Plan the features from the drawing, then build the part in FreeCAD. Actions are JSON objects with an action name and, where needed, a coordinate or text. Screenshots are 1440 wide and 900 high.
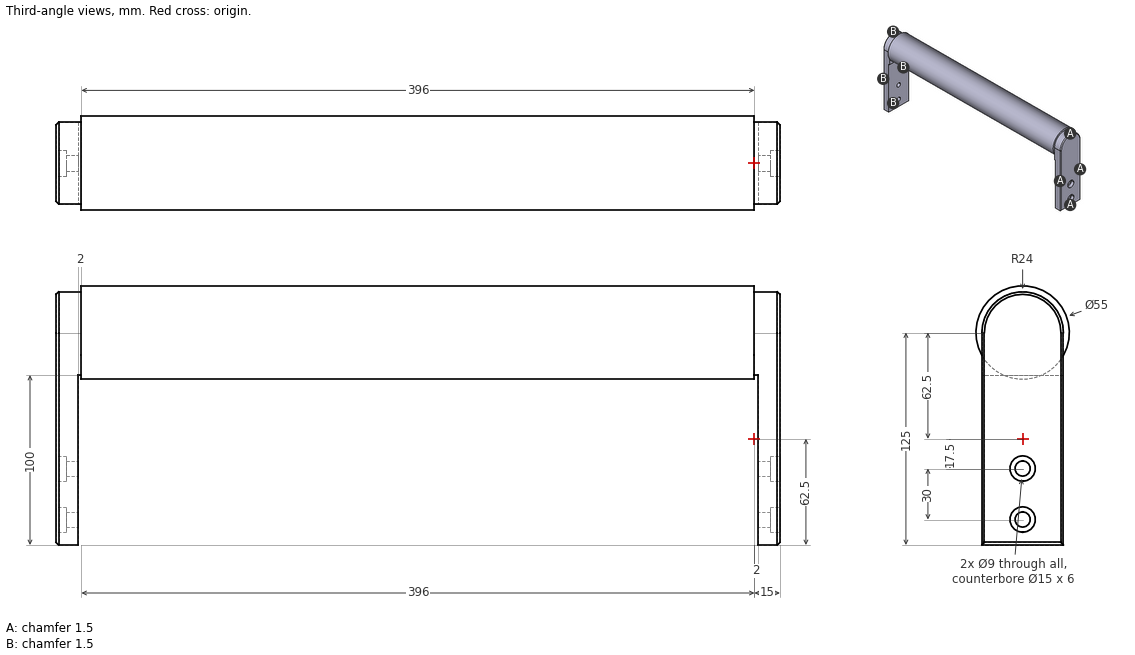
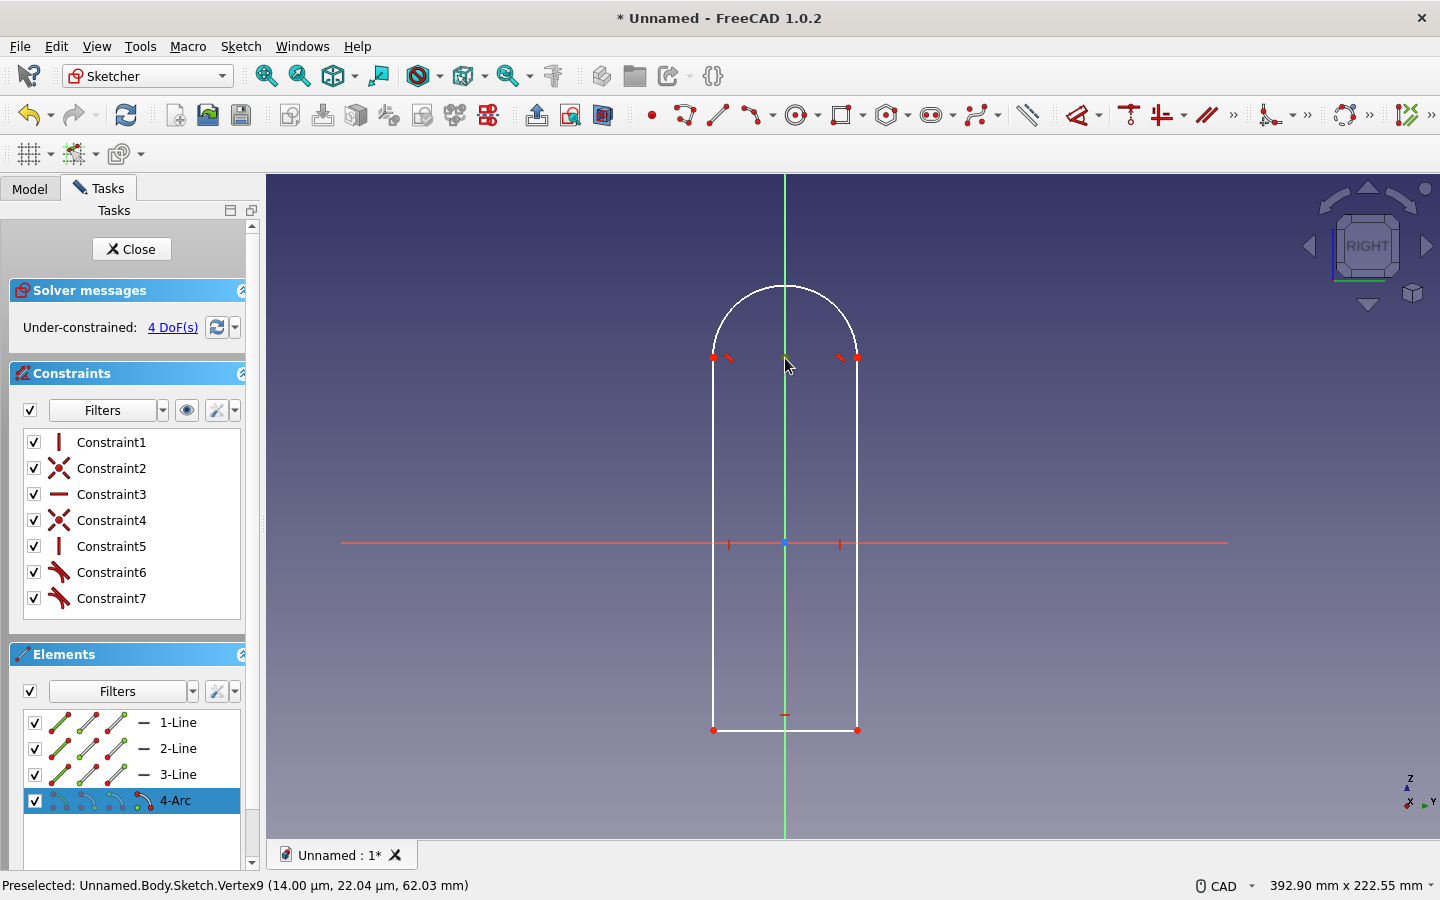
{"action": "left_click", "coordinate": [785, 768]}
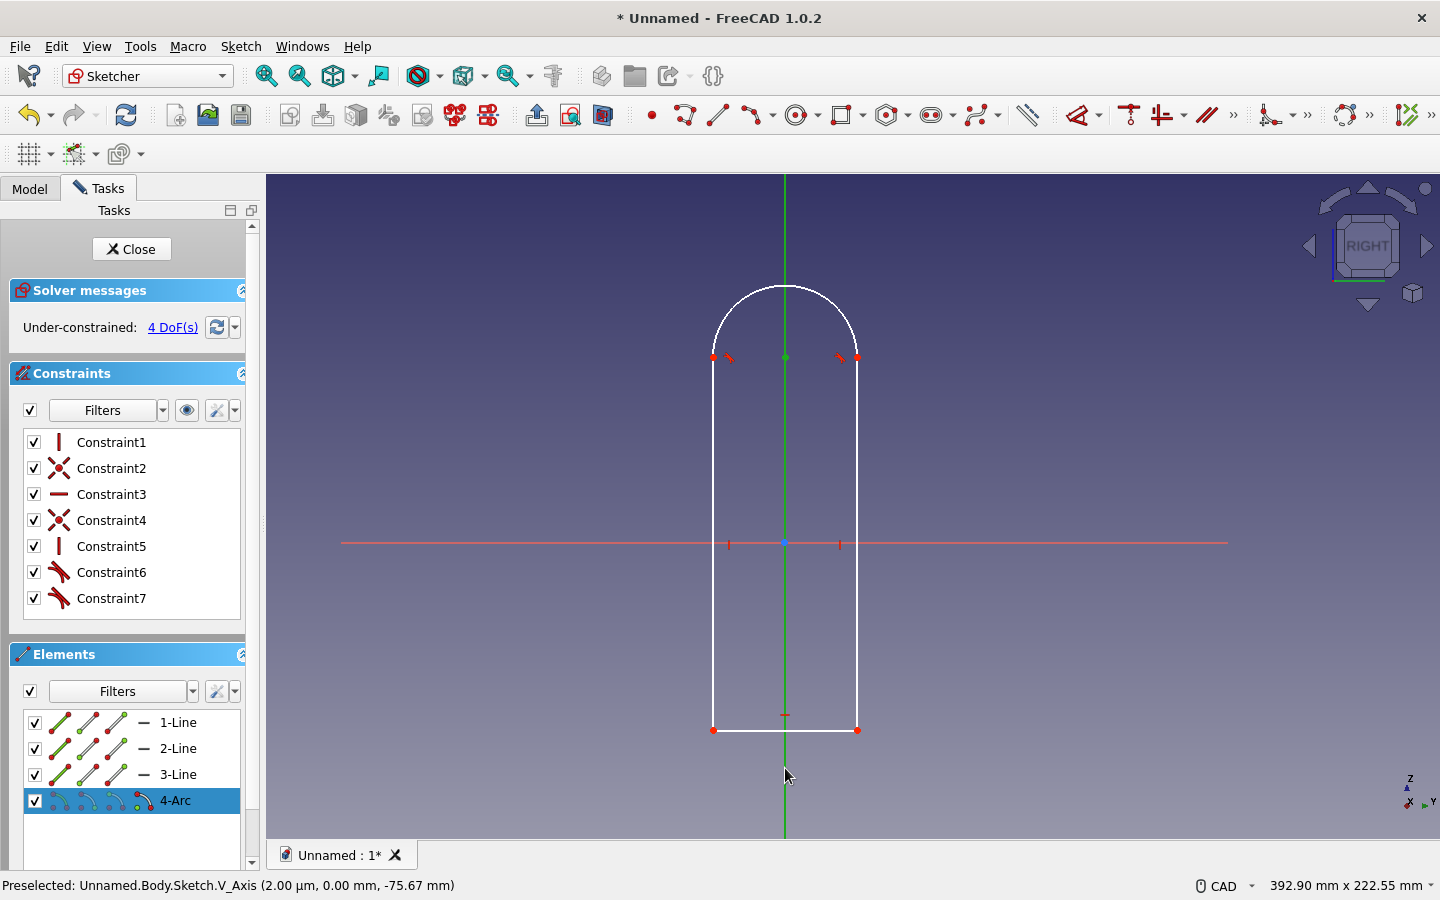
{"action": "left_click", "coordinate": [1129, 116]}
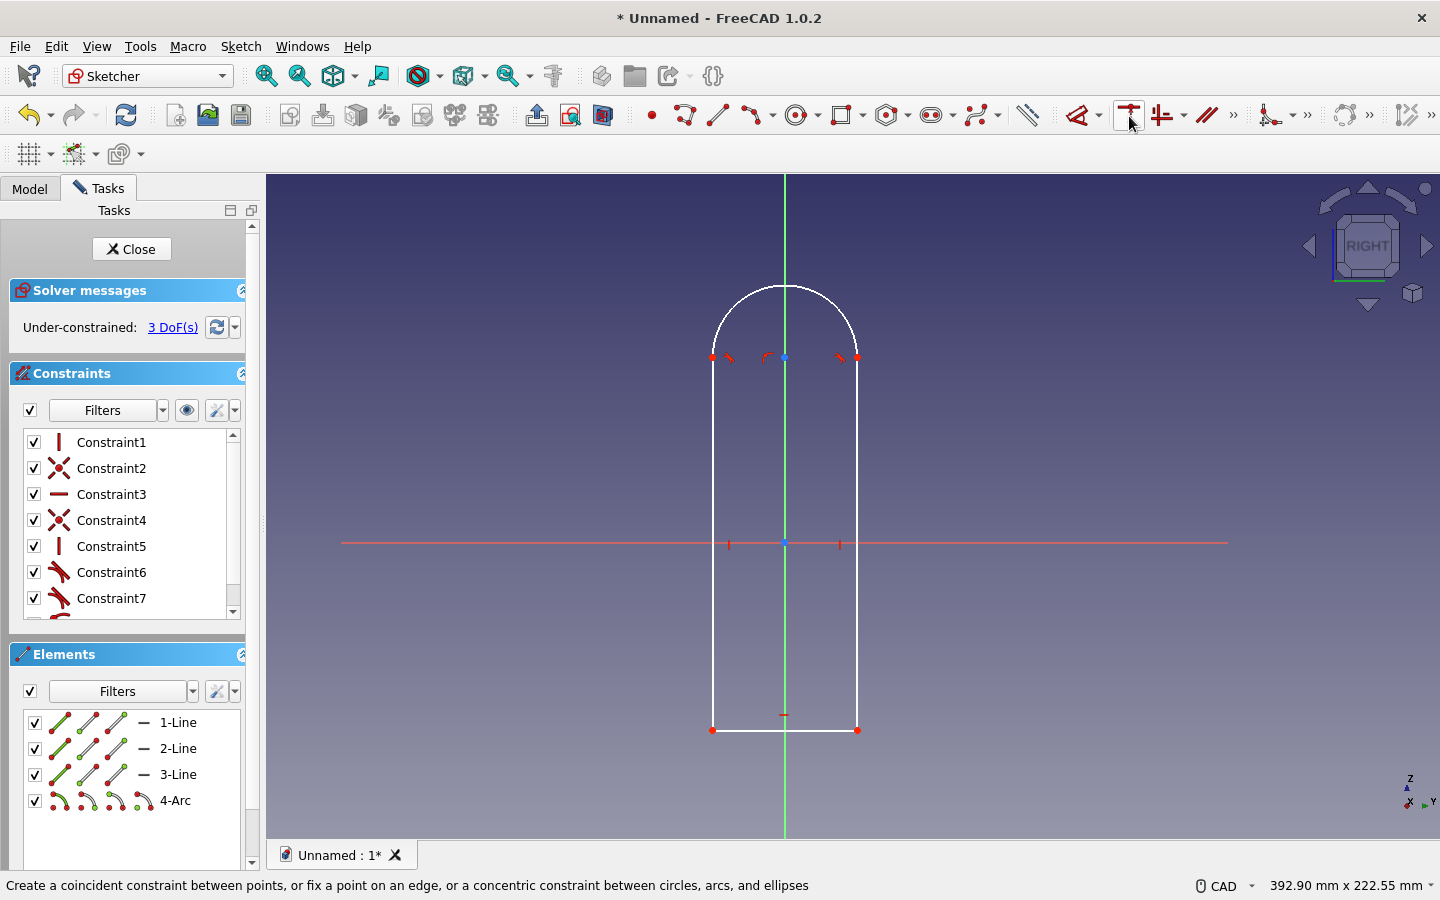
{"action": "left_click", "coordinate": [1076, 116]}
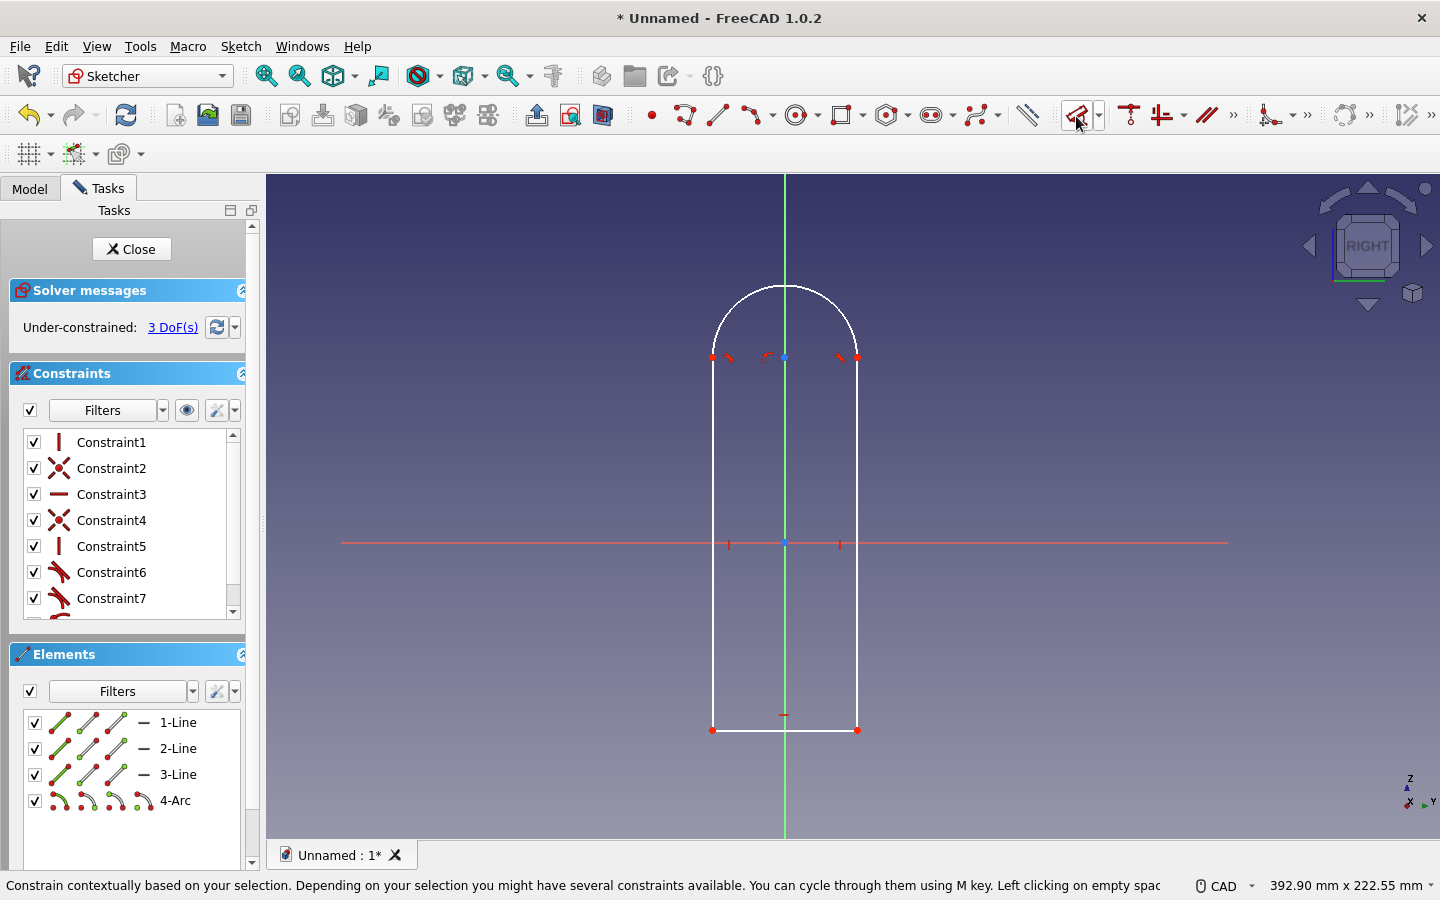
{"action": "left_click", "coordinate": [827, 299]}
{"action": "left_click", "coordinate": [846, 273]}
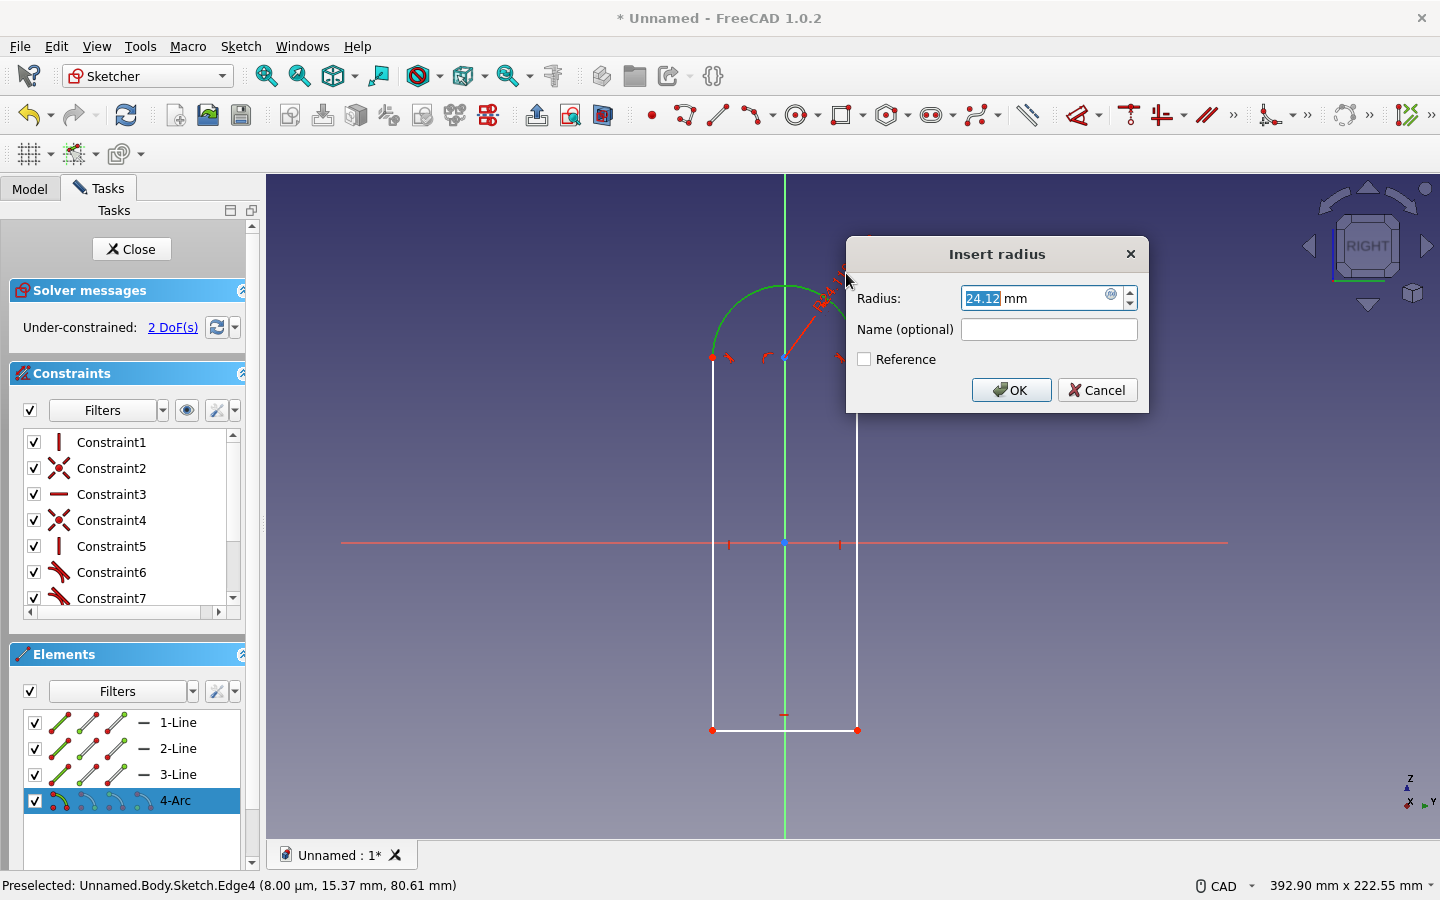
{"action": "type", "text": "24"}
{"action": "key", "text": "Return"}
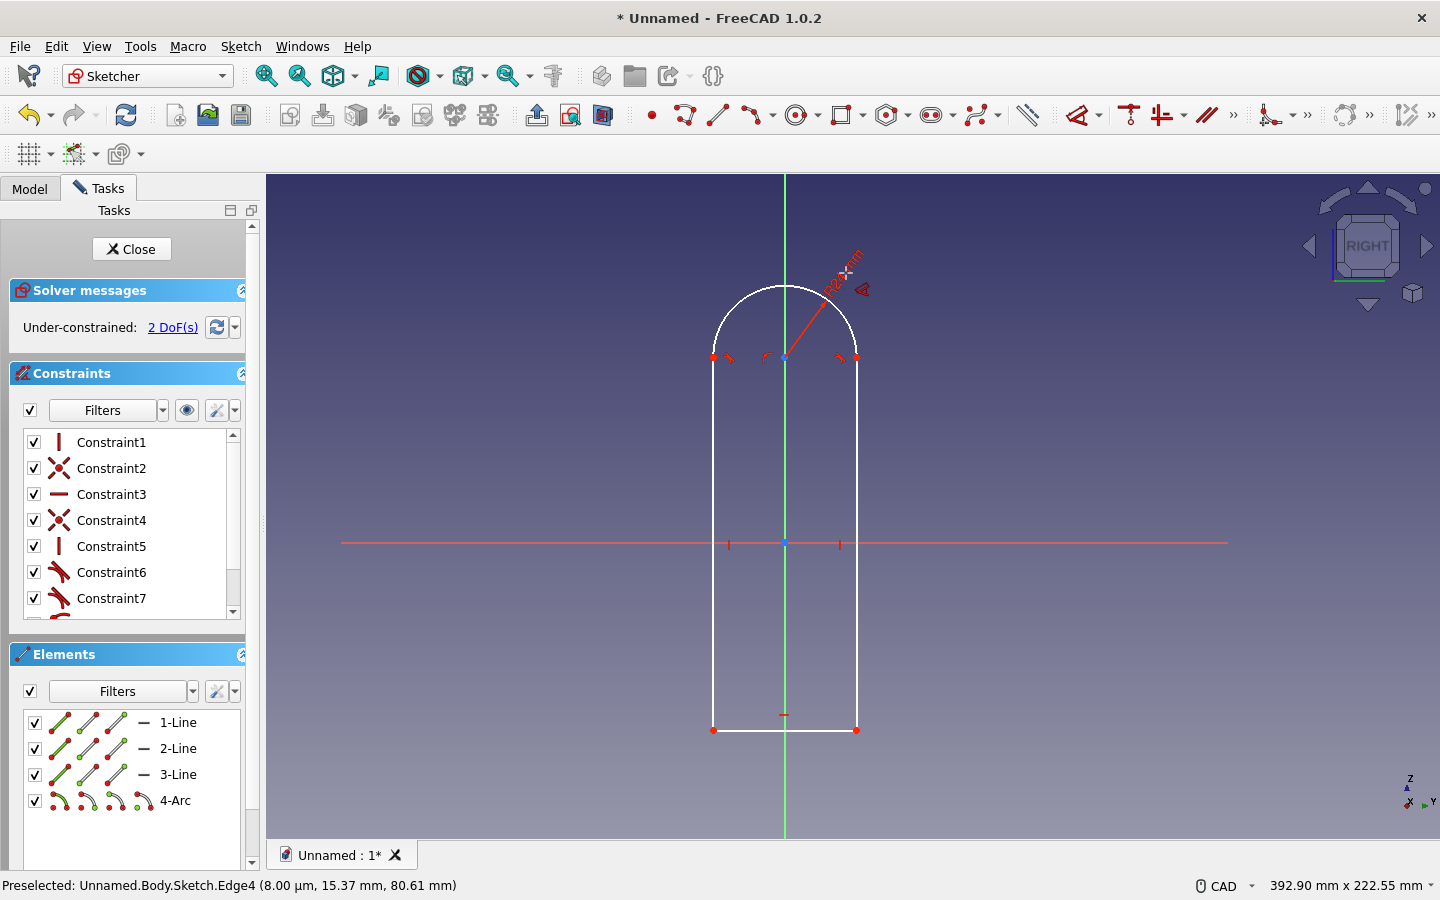
{"action": "left_click", "coordinate": [713, 470]}
{"action": "left_click", "coordinate": [679, 458]}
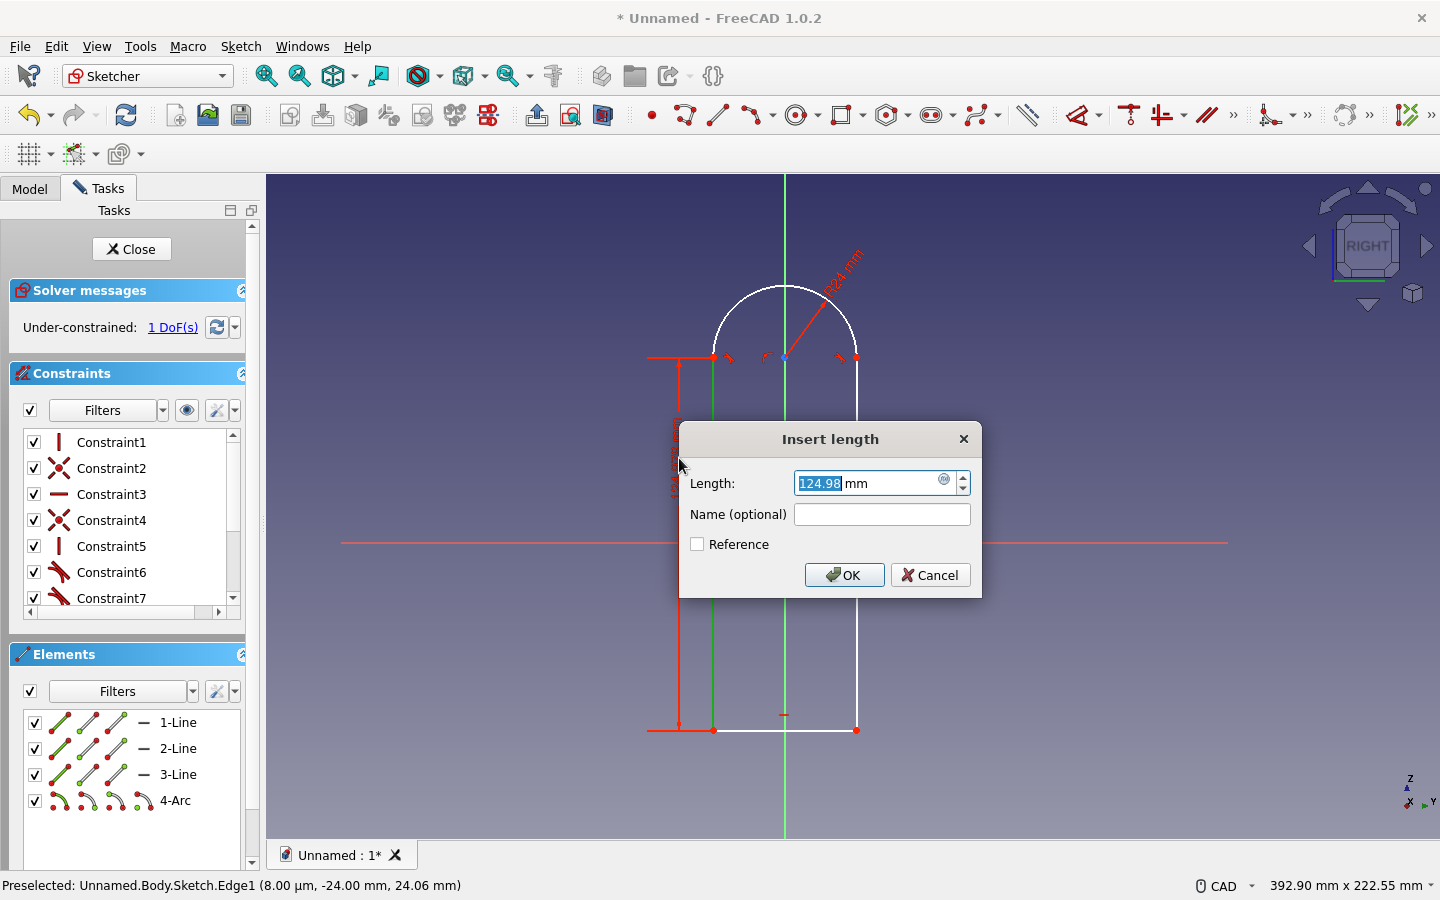
{"action": "type", "text": "125"}
{"action": "key", "text": "Return"}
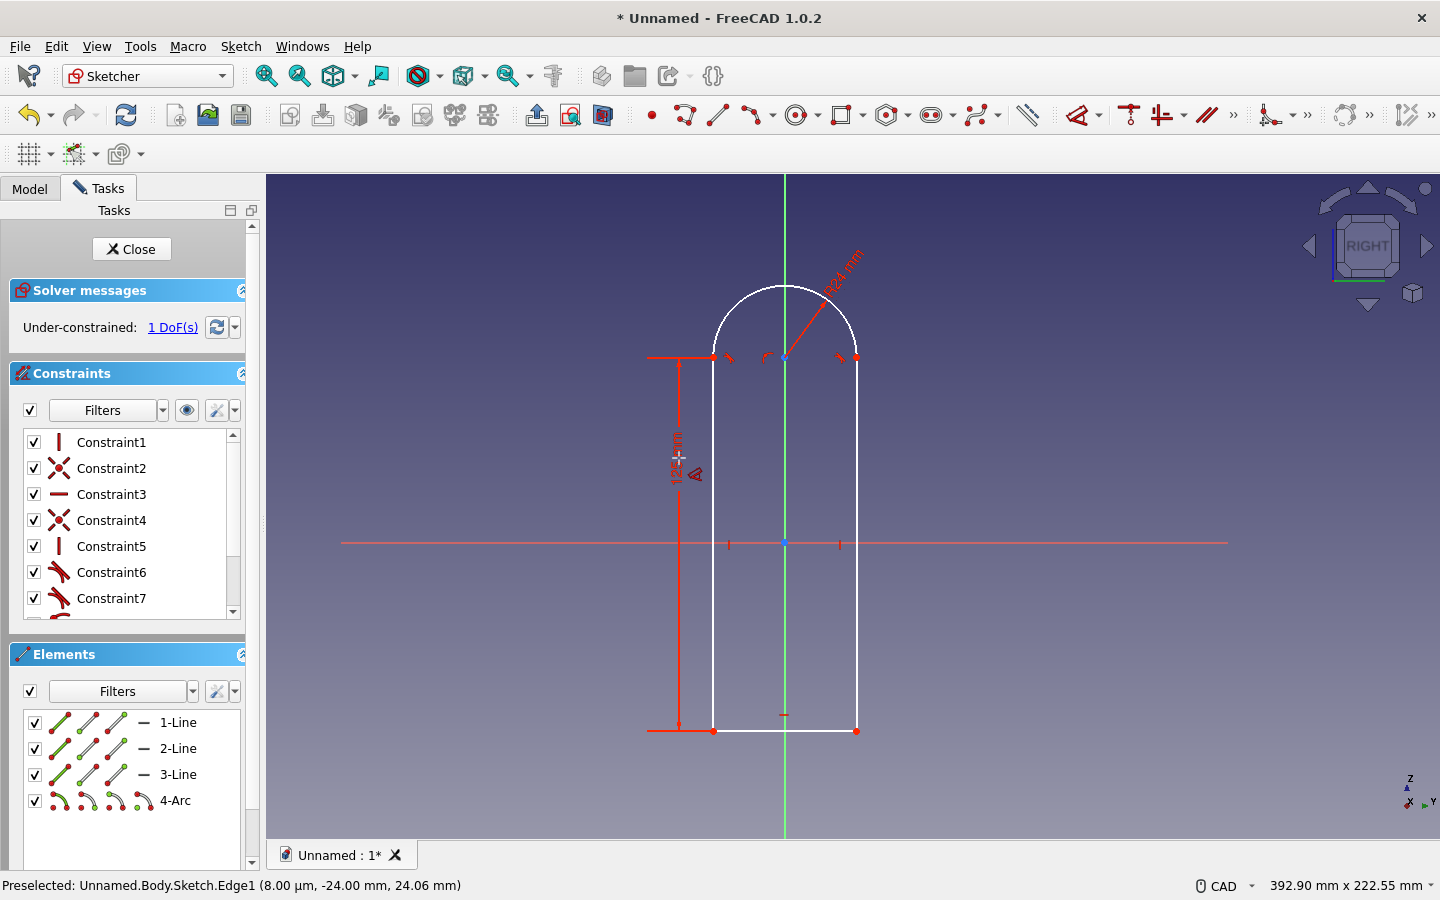
{"action": "left_click", "coordinate": [713, 358]}
{"action": "left_click", "coordinate": [679, 408]}